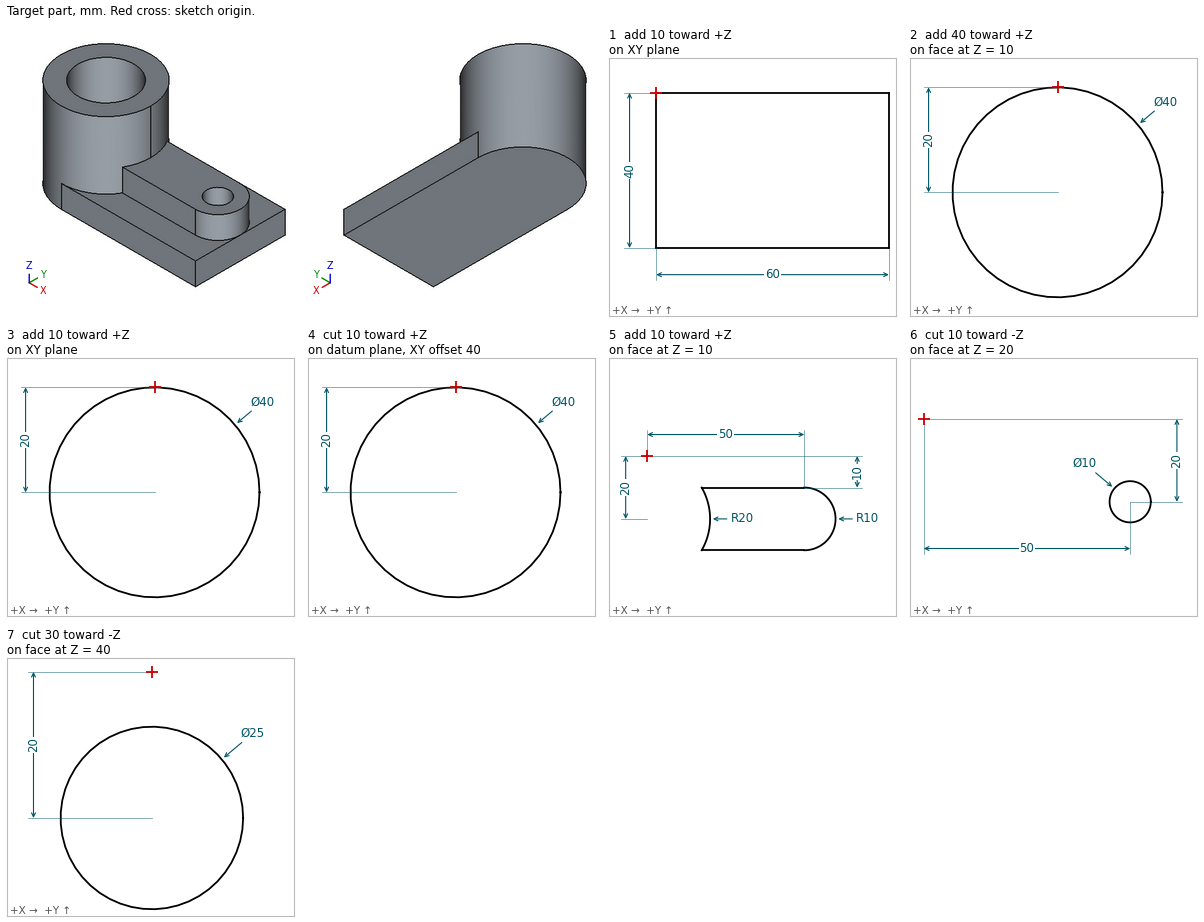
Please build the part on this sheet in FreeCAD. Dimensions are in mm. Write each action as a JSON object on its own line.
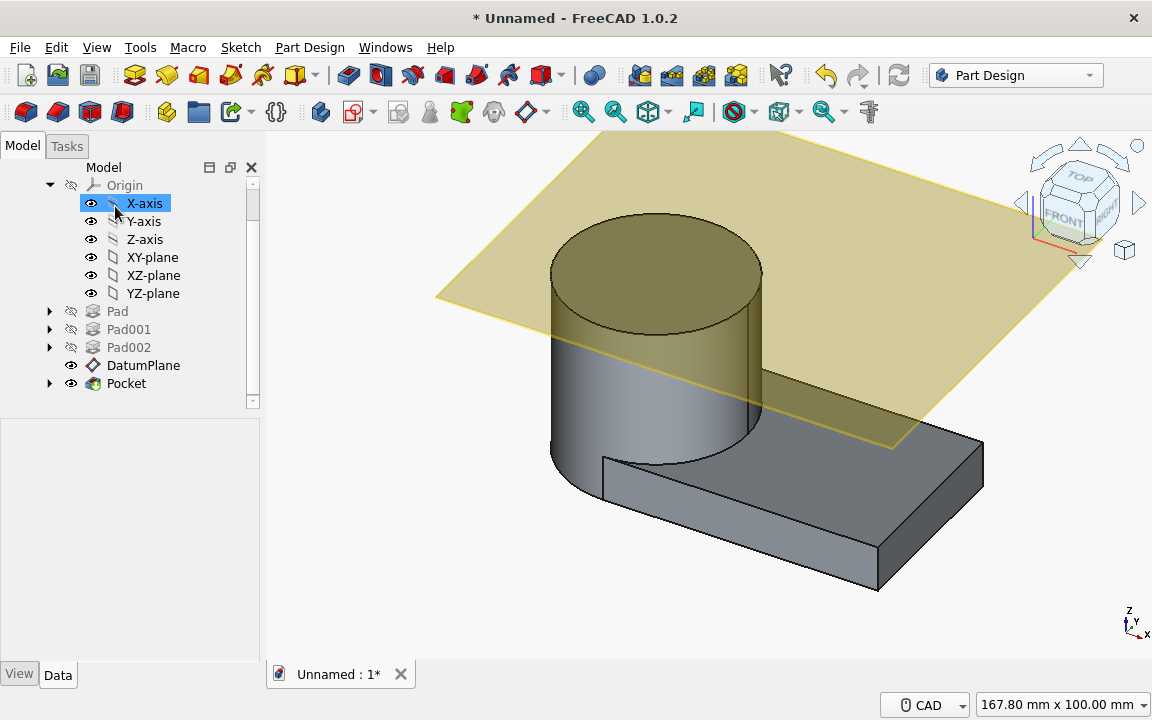
{"action": "left_click", "coordinate": [116, 365]}
{"action": "key", "text": "space"}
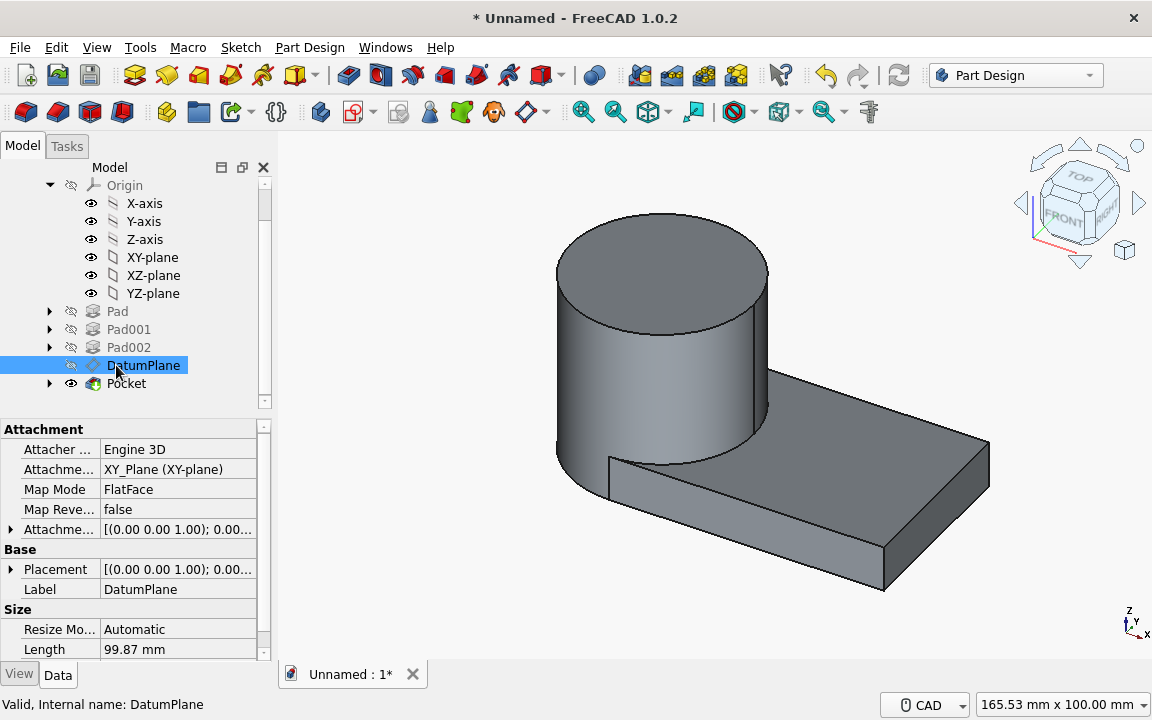
{"action": "left_click", "coordinate": [839, 462]}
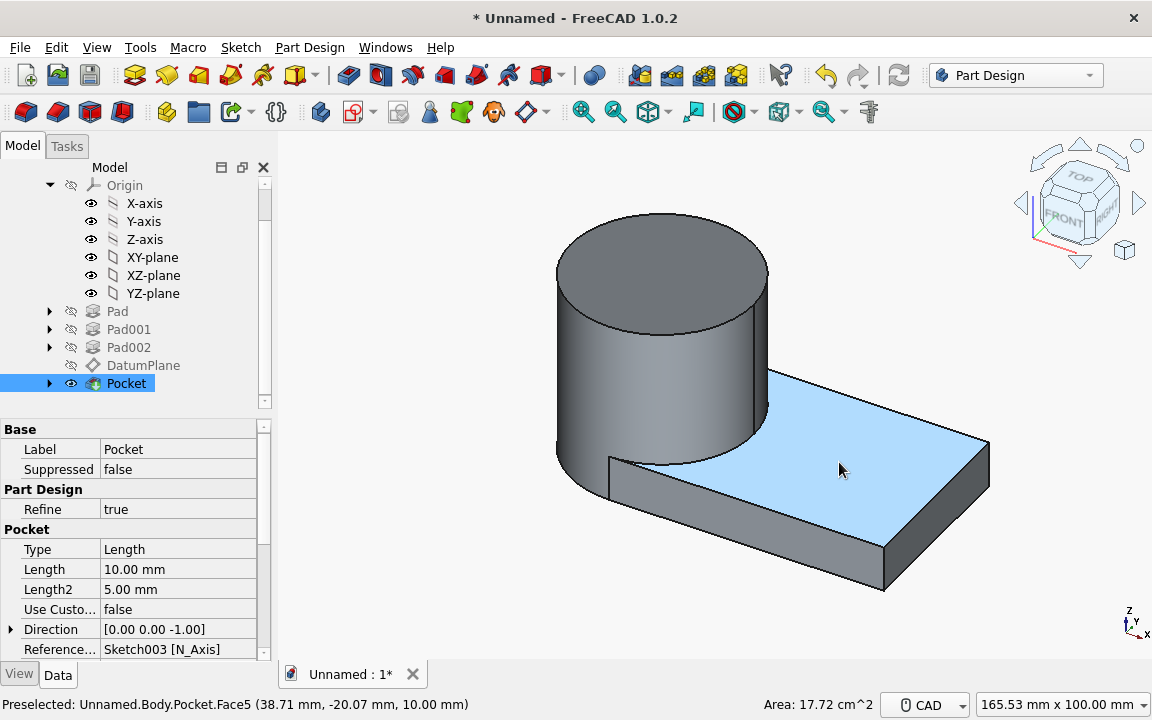
{"action": "left_click", "coordinate": [354, 112]}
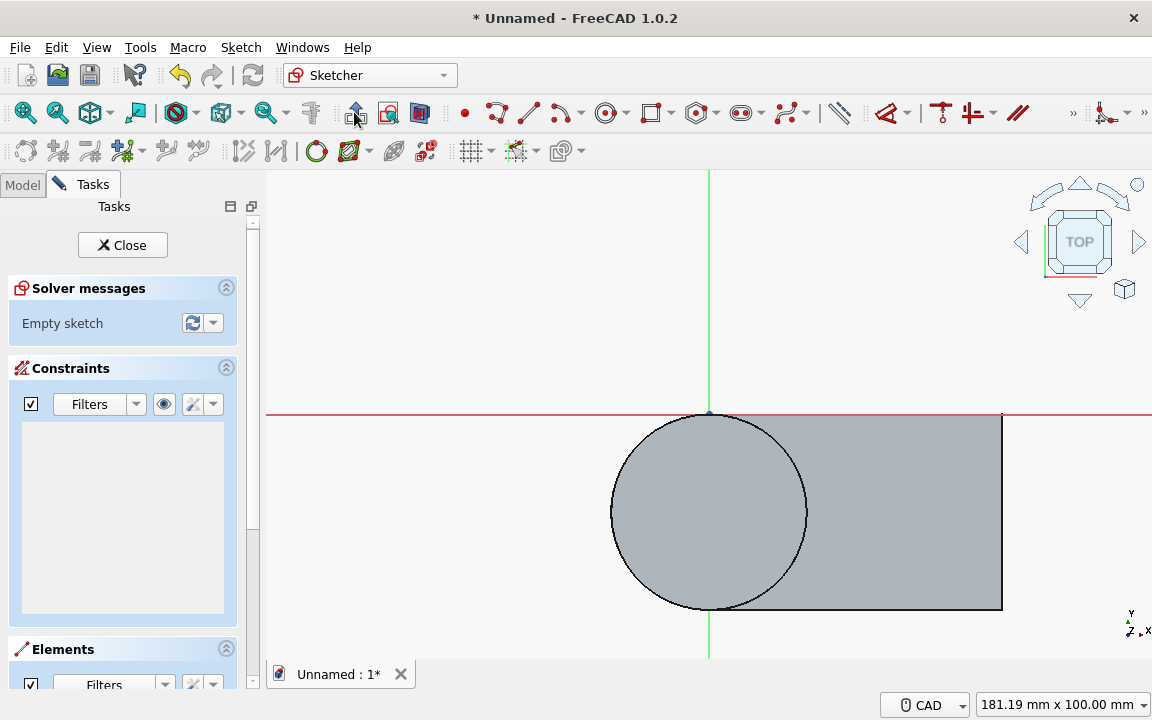
{"action": "scroll", "coordinate": [640, 414], "scroll_direction": "down", "scroll_amount": 5}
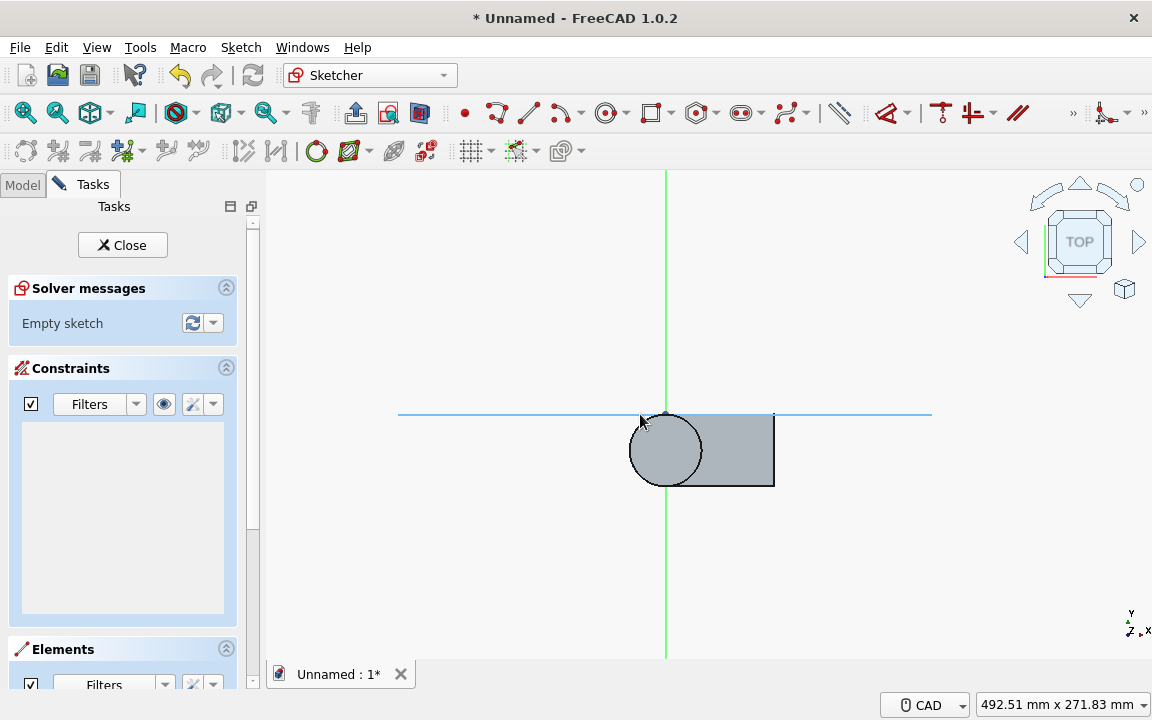
{"action": "scroll", "coordinate": [740, 448], "scroll_direction": "up", "scroll_amount": 8}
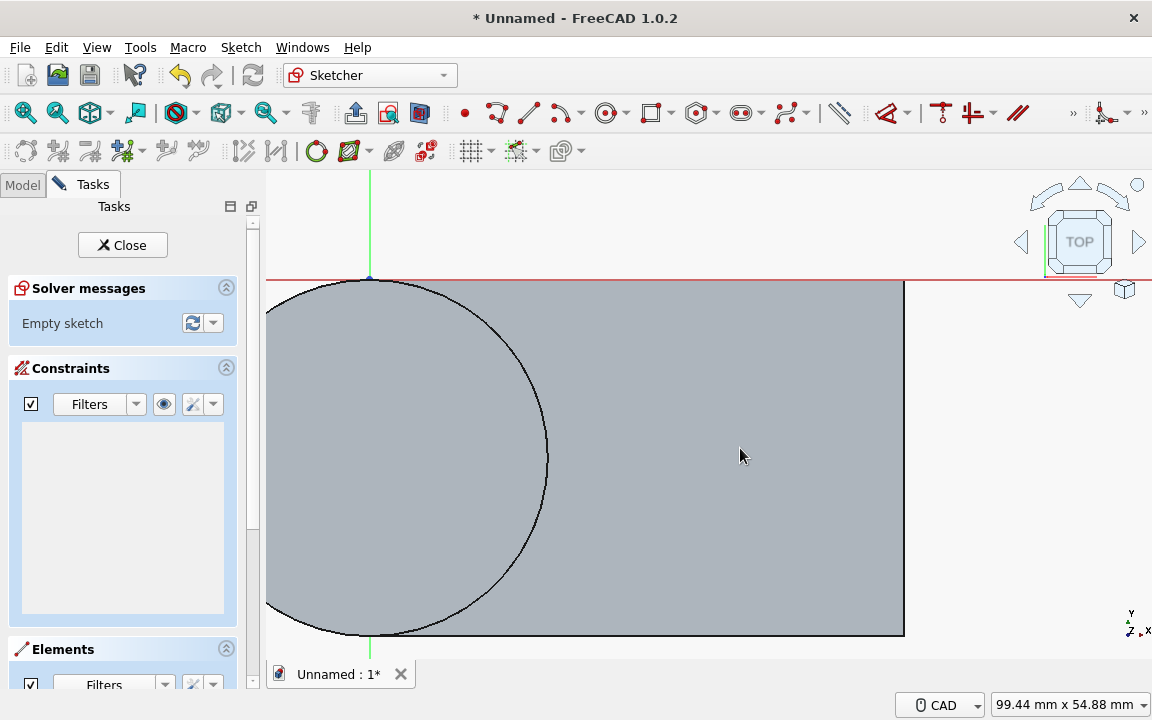
{"action": "left_click", "coordinate": [530, 114]}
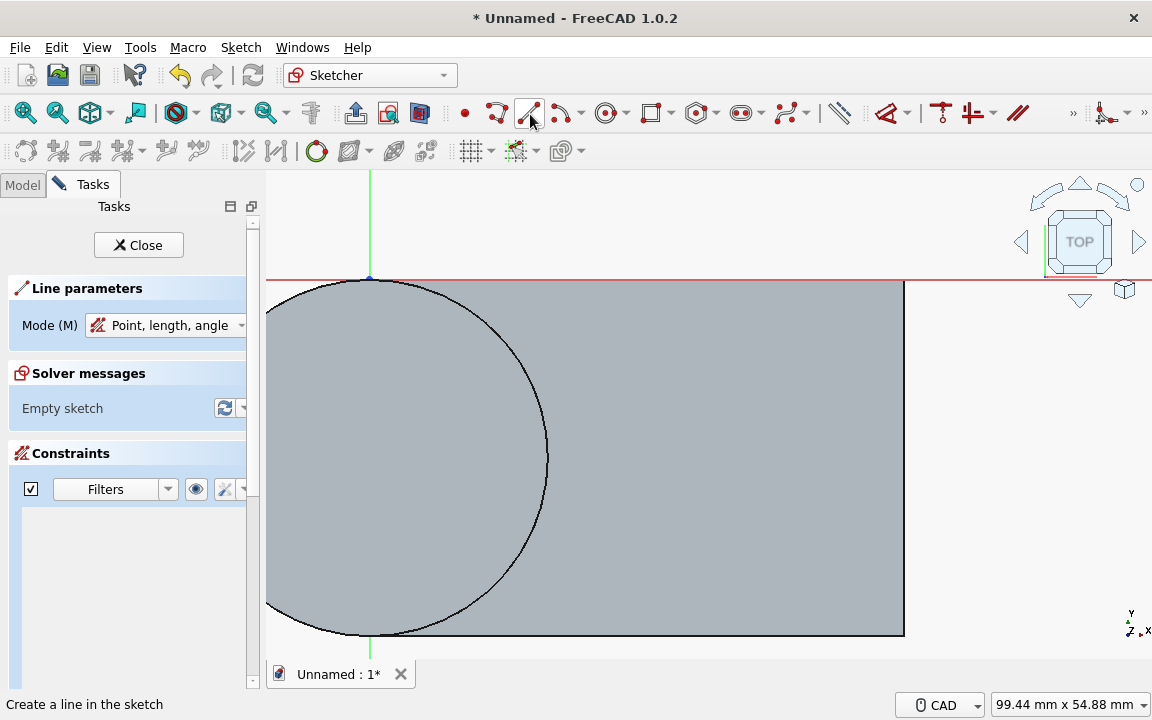
{"action": "left_click", "coordinate": [815, 369]}
{"action": "left_click", "coordinate": [524, 369]}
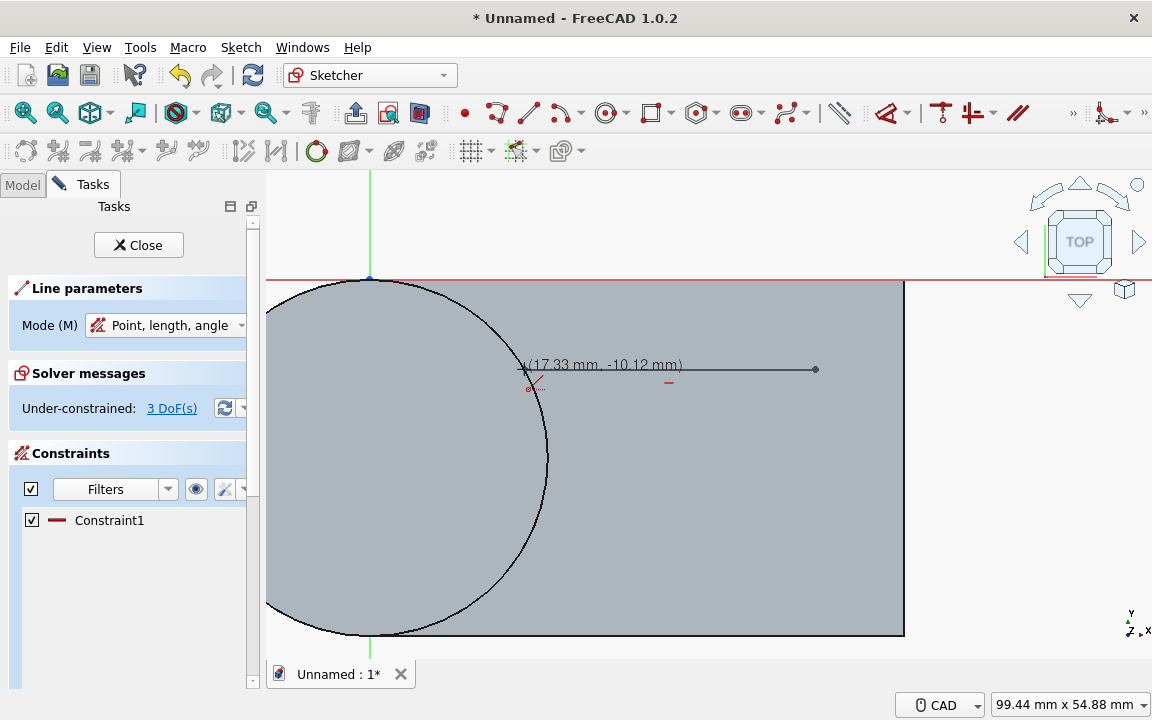
{"action": "left_click", "coordinate": [524, 547]}
{"action": "left_click", "coordinate": [815, 547]}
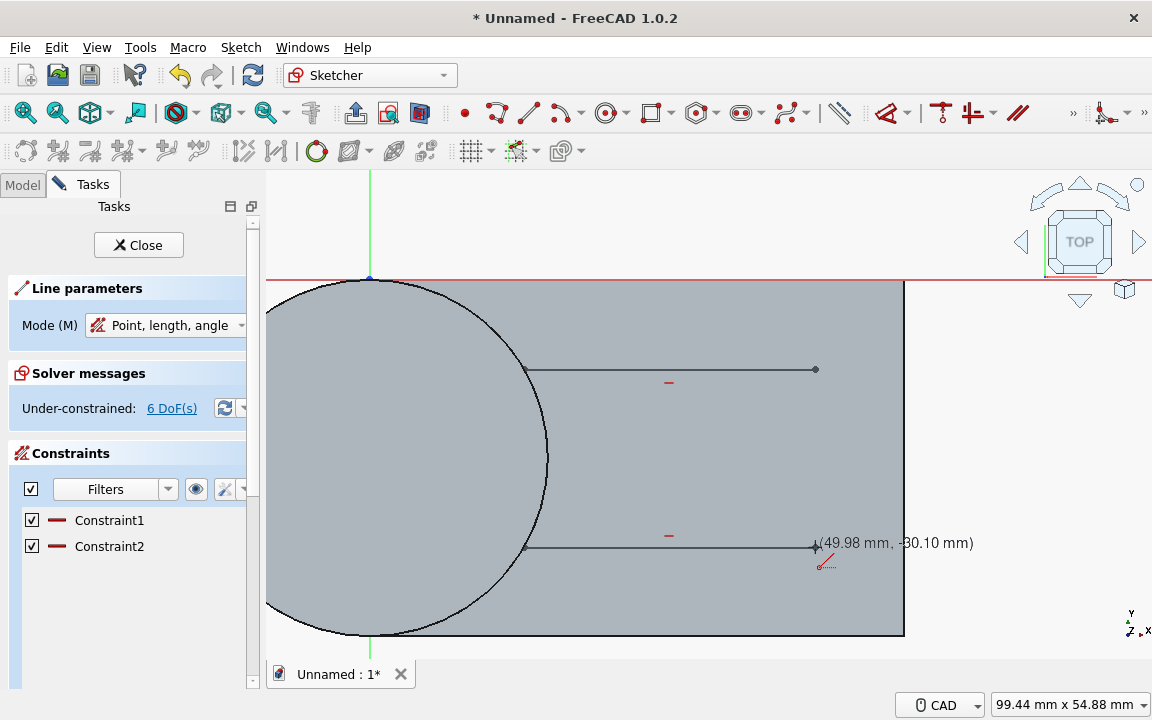
{"action": "left_click", "coordinate": [584, 114]}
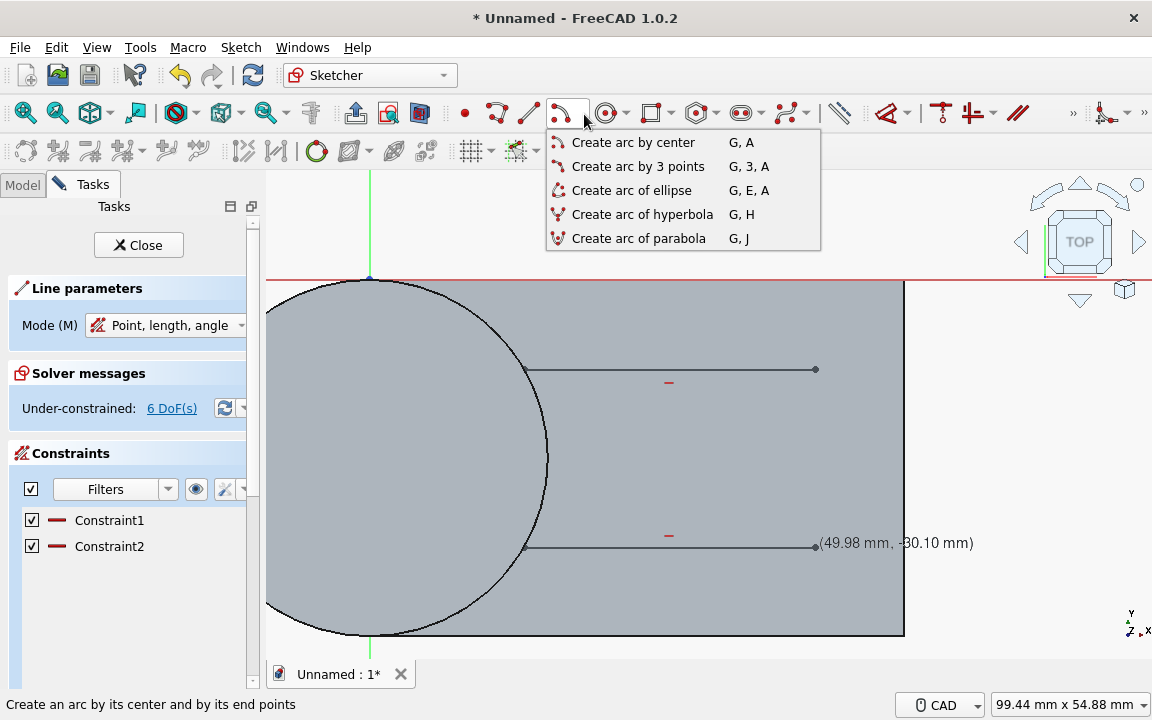
{"action": "left_click", "coordinate": [684, 166]}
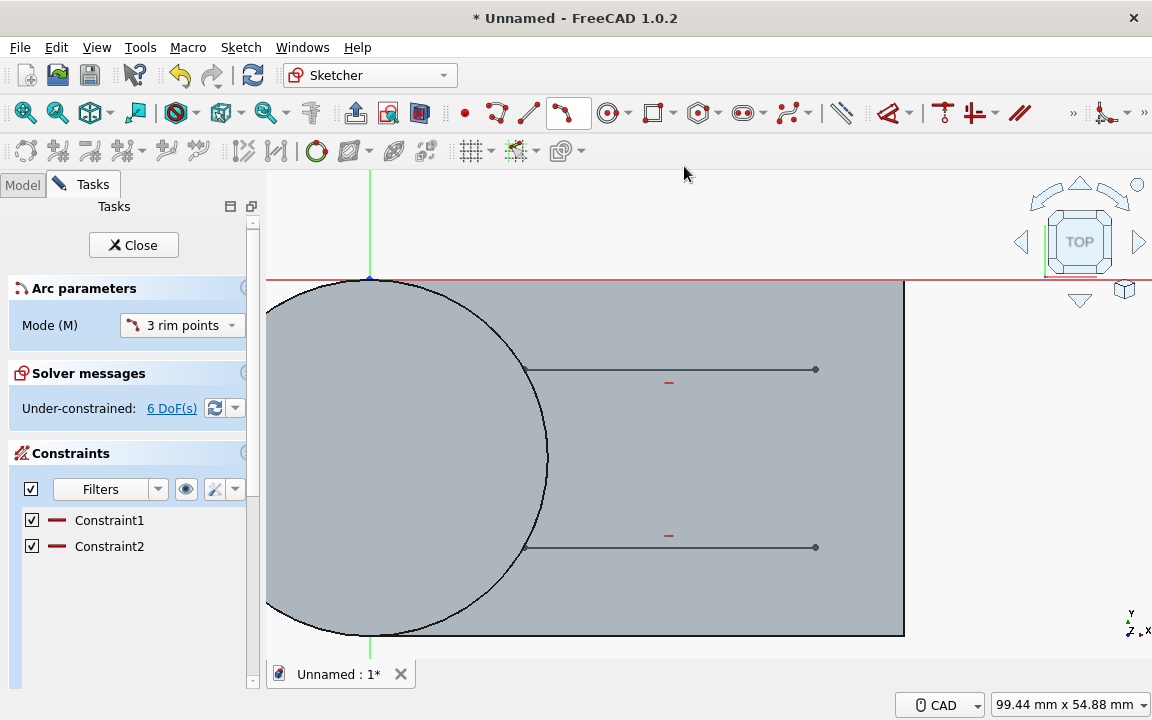
{"action": "left_click", "coordinate": [524, 370]}
{"action": "left_click", "coordinate": [524, 548]}
{"action": "left_click", "coordinate": [548, 458]}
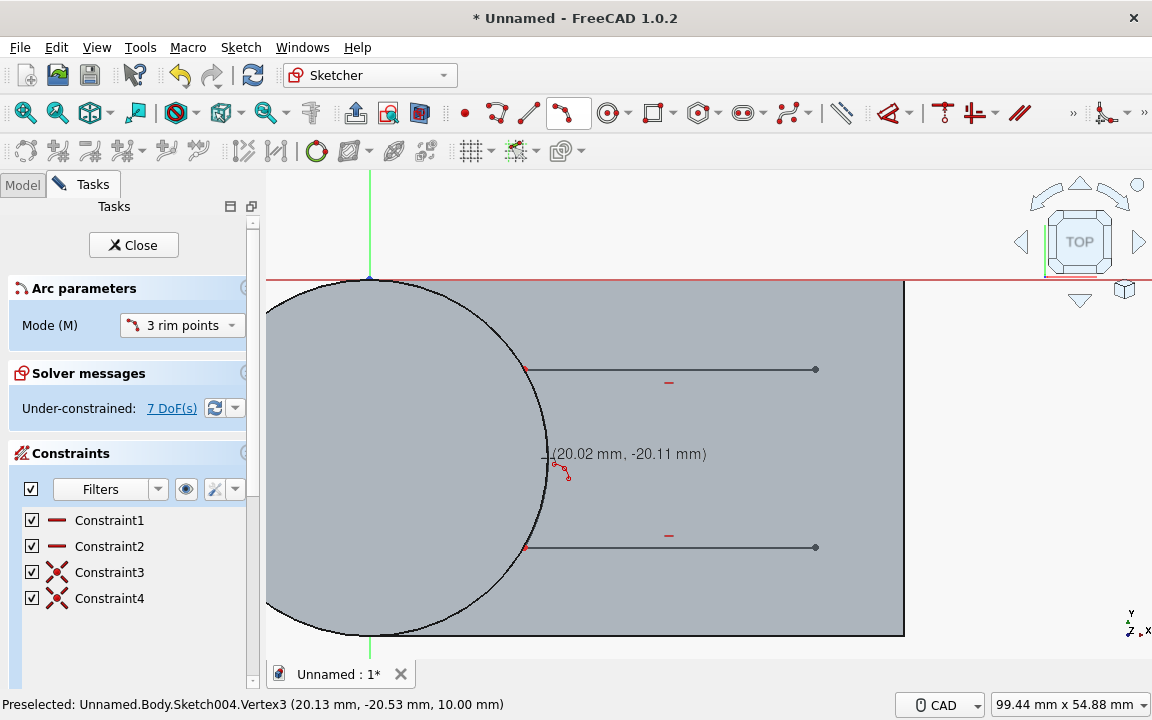
{"action": "left_click", "coordinate": [815, 548]}
{"action": "left_click", "coordinate": [815, 370]}
{"action": "left_click", "coordinate": [904, 458]}
{"action": "key", "text": "Escape"}